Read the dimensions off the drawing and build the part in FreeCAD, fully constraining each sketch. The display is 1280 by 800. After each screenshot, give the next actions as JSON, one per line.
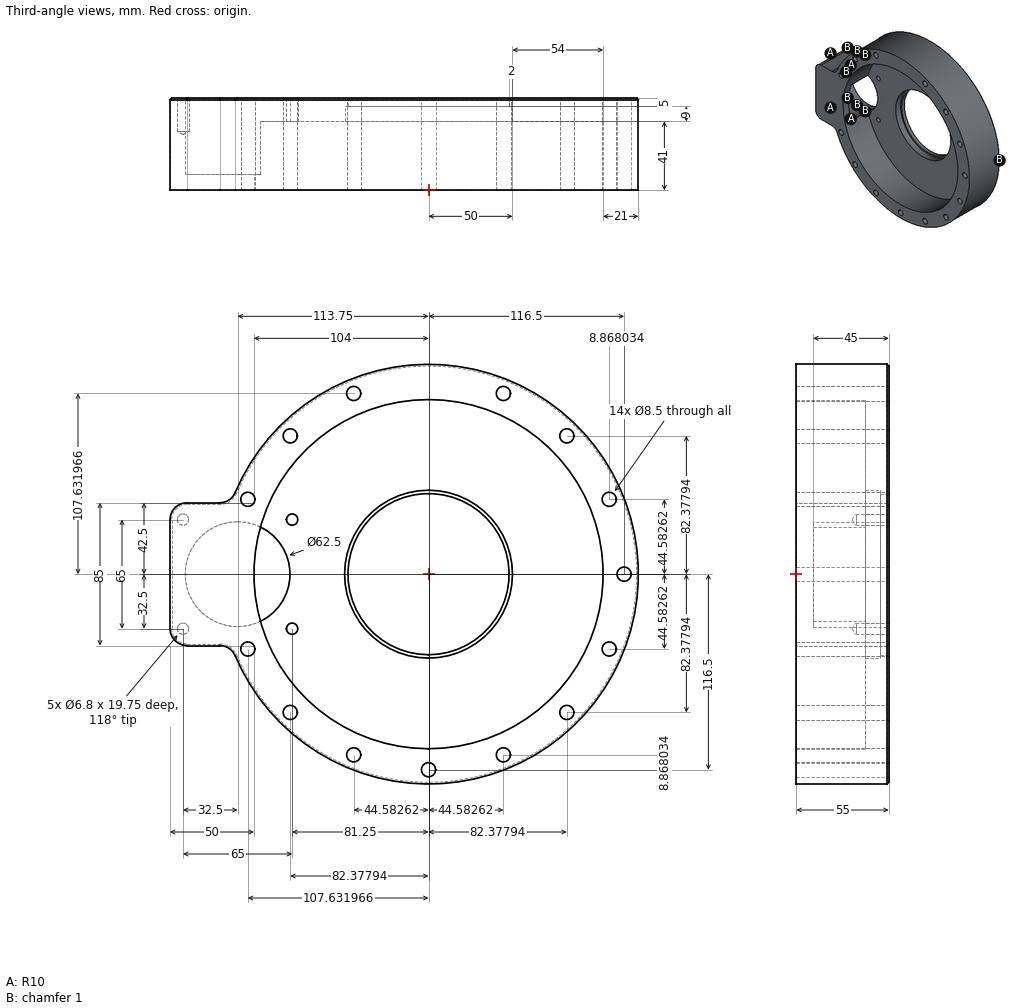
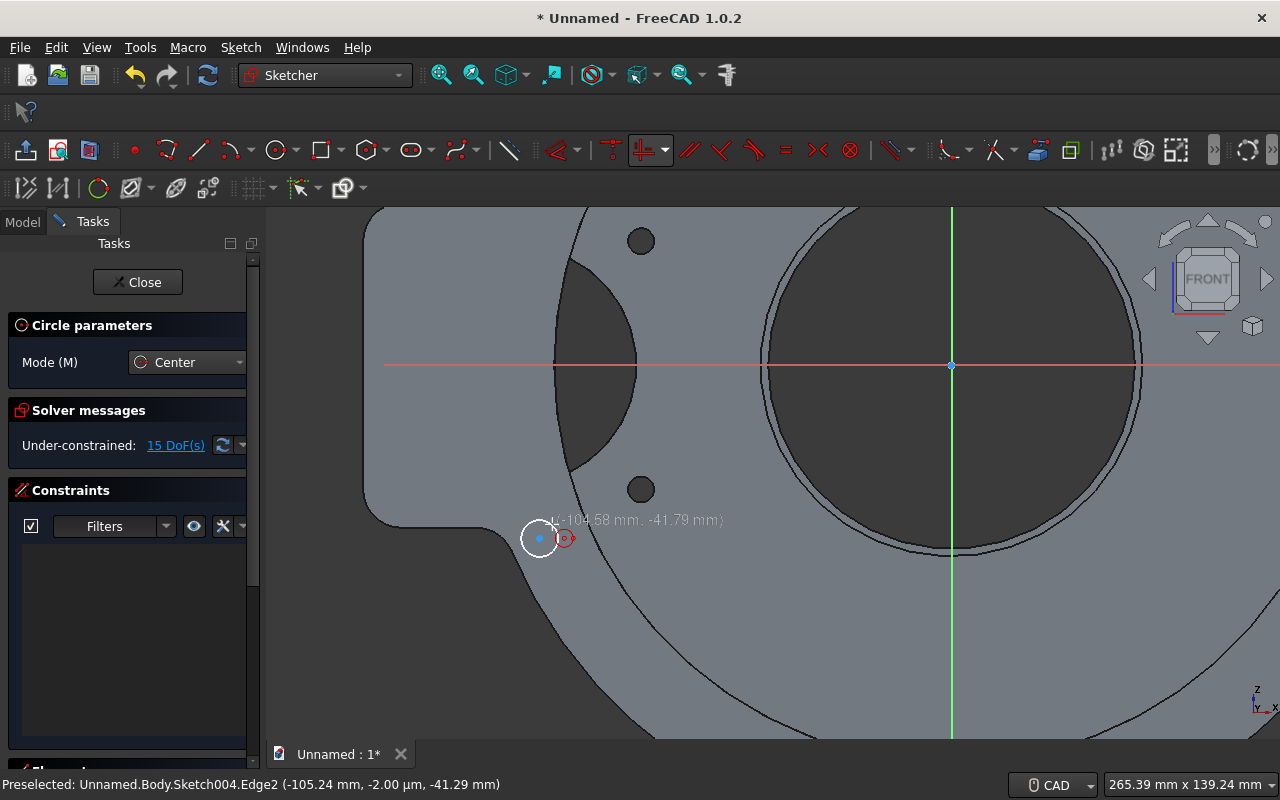
{"action": "scroll", "coordinate": [551, 526], "scroll_direction": "down", "scroll_amount": 5}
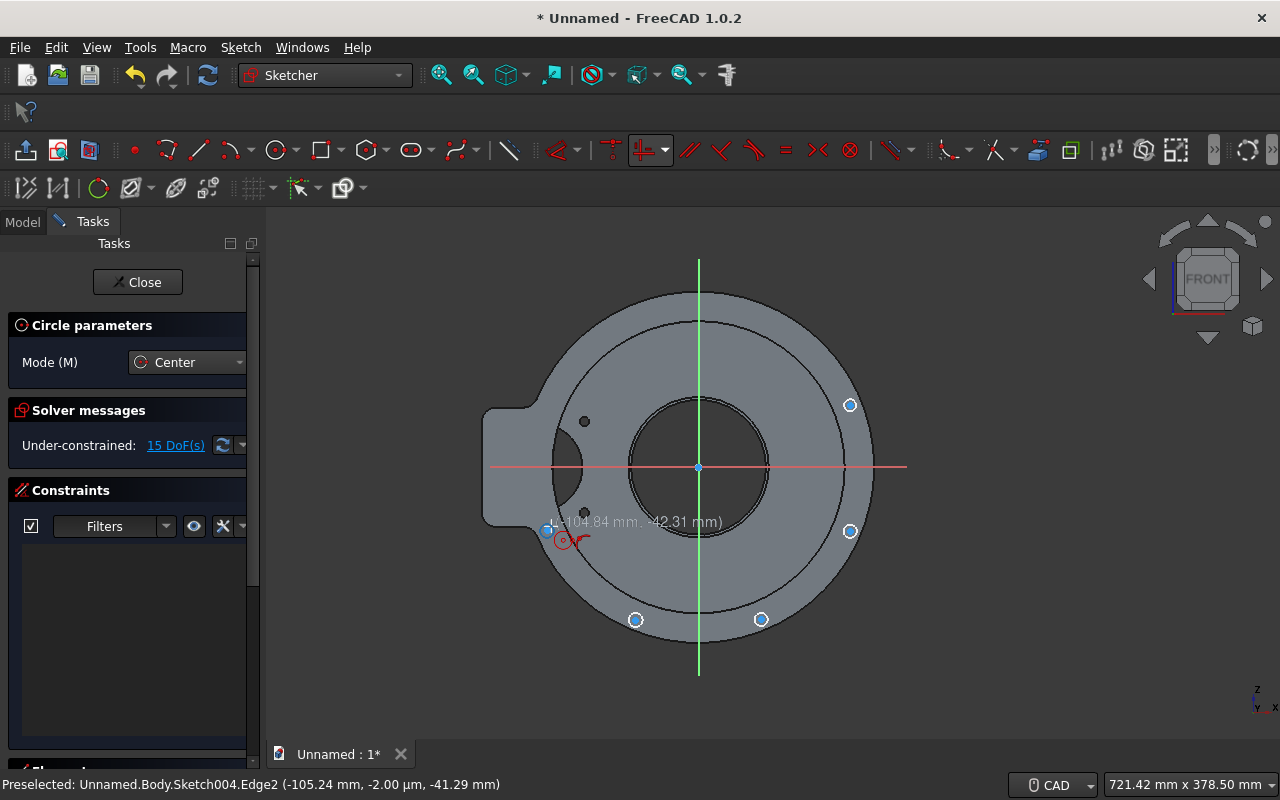
{"action": "scroll", "coordinate": [547, 405], "scroll_direction": "up", "scroll_amount": 7}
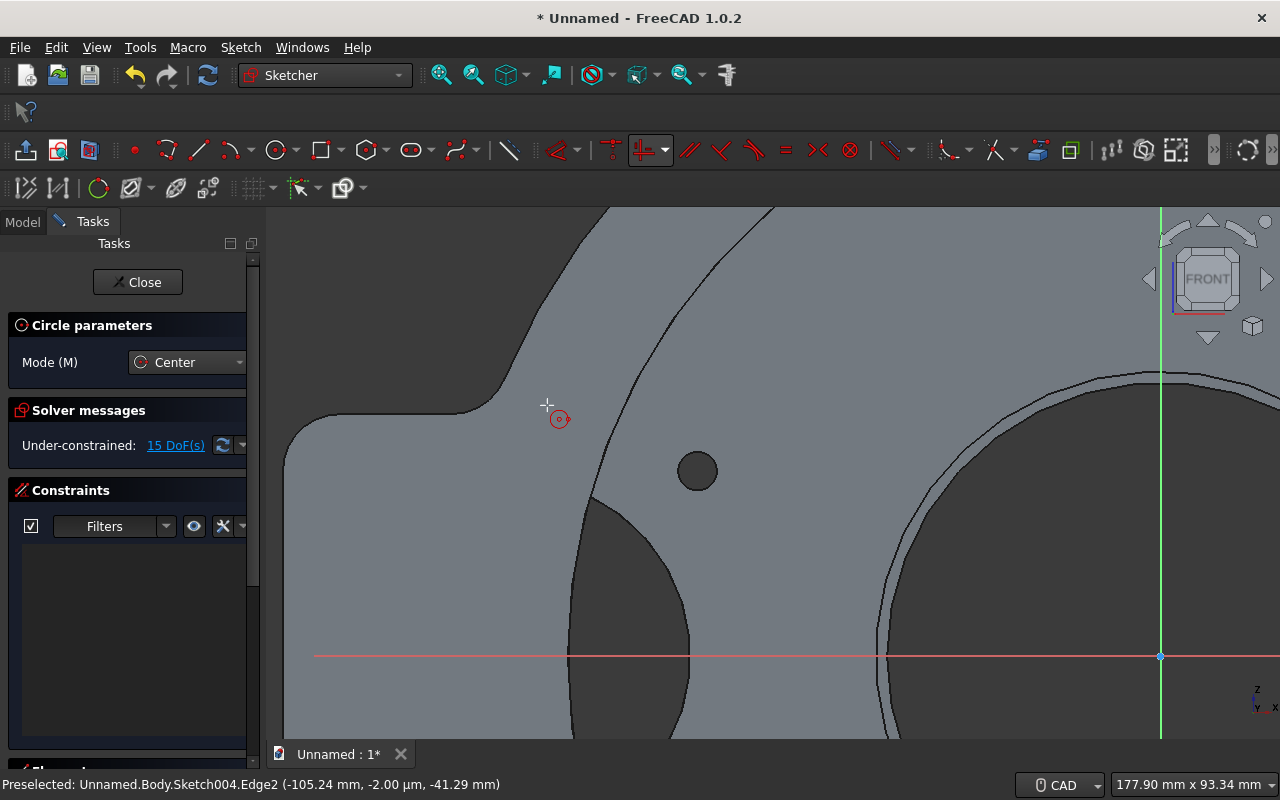
{"action": "scroll", "coordinate": [547, 405], "scroll_direction": "down", "scroll_amount": 7}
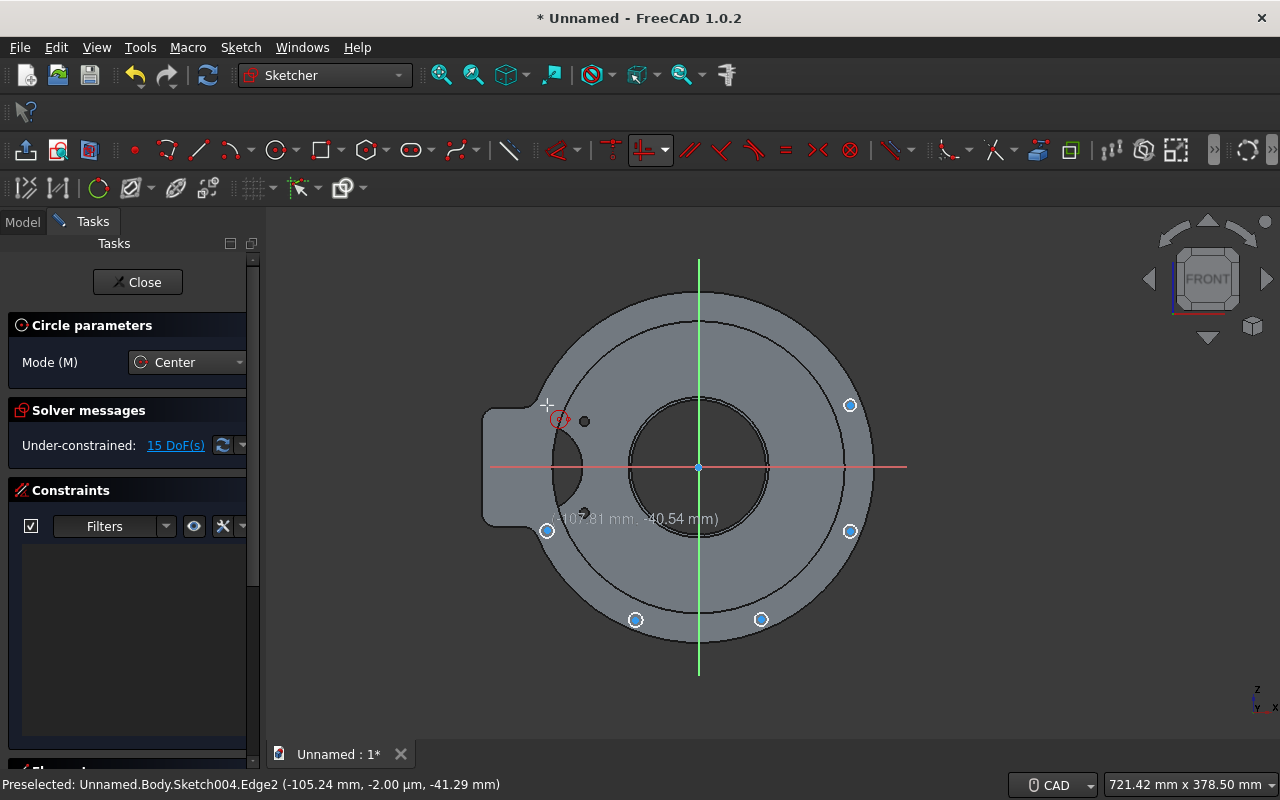
{"action": "left_click", "coordinate": [547, 405]}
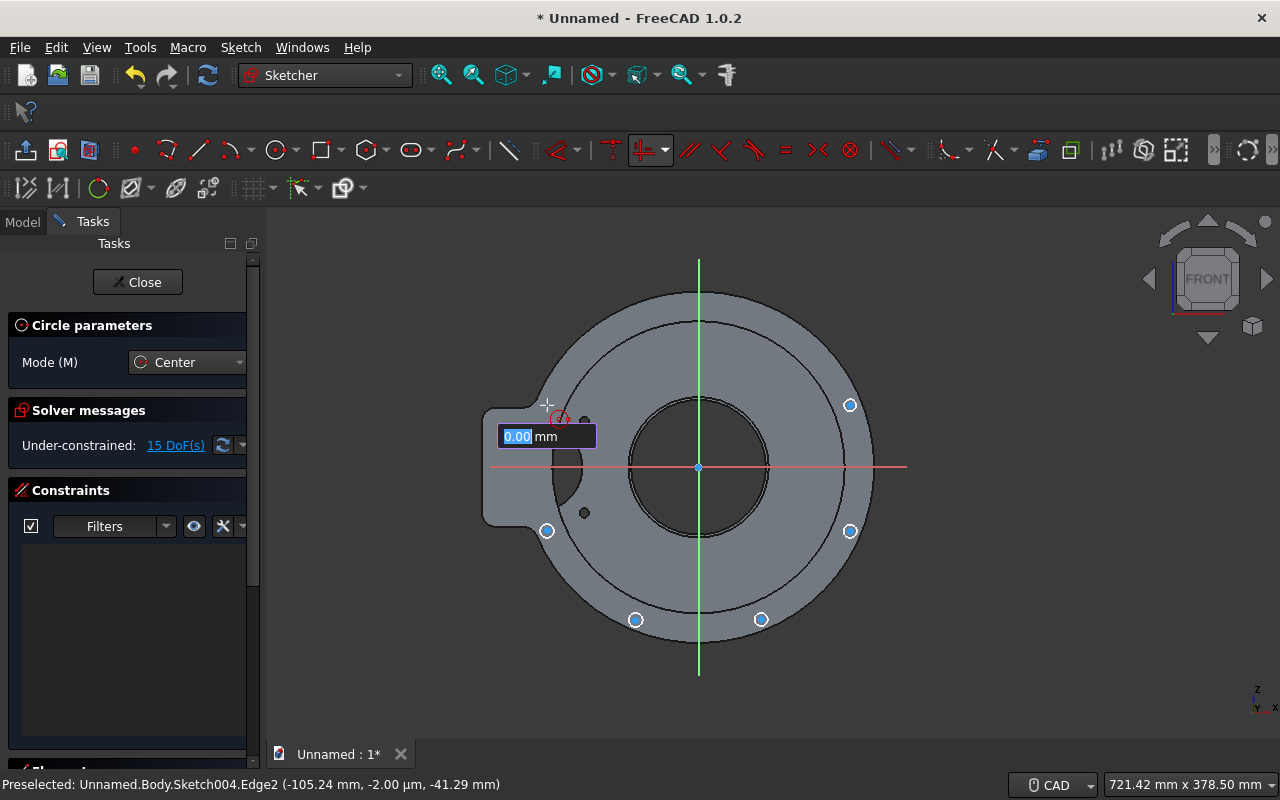
{"action": "scroll", "coordinate": [551, 400], "scroll_direction": "up", "scroll_amount": 5}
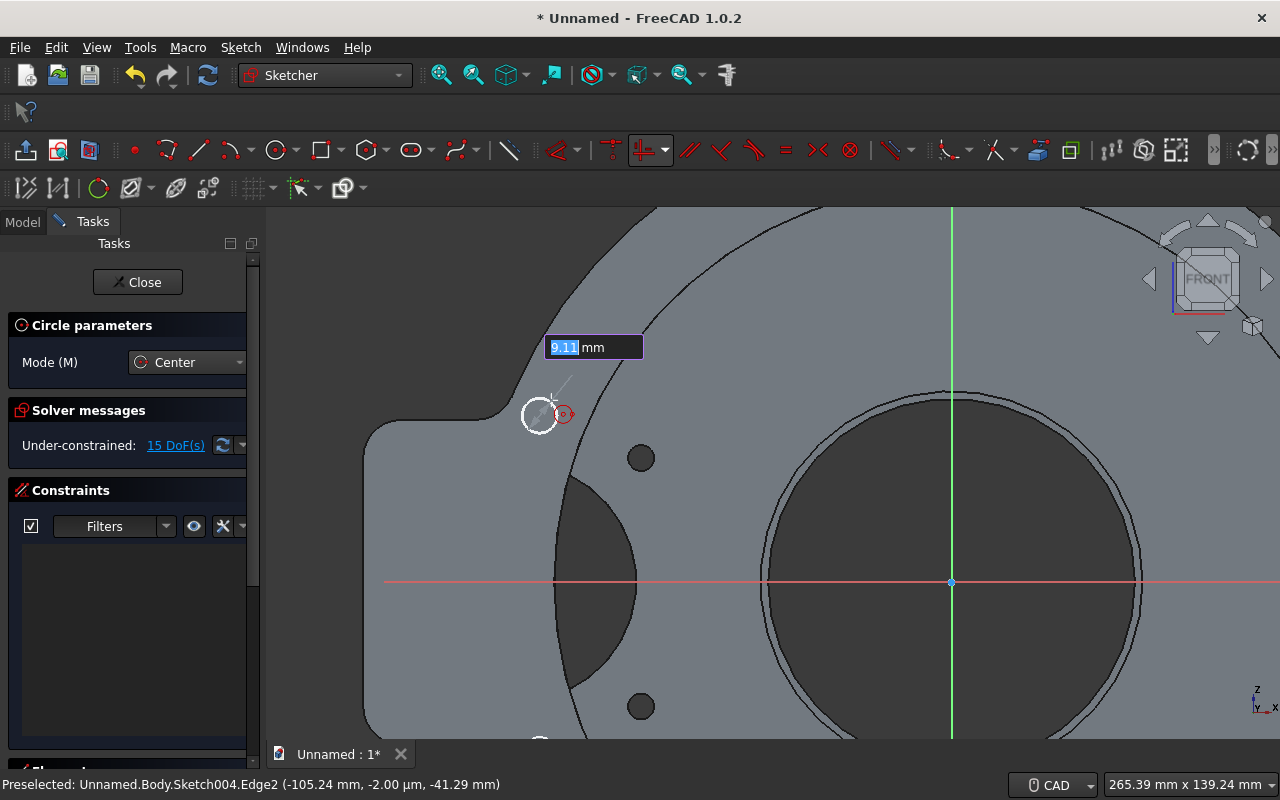
{"action": "left_click", "coordinate": [552, 400]}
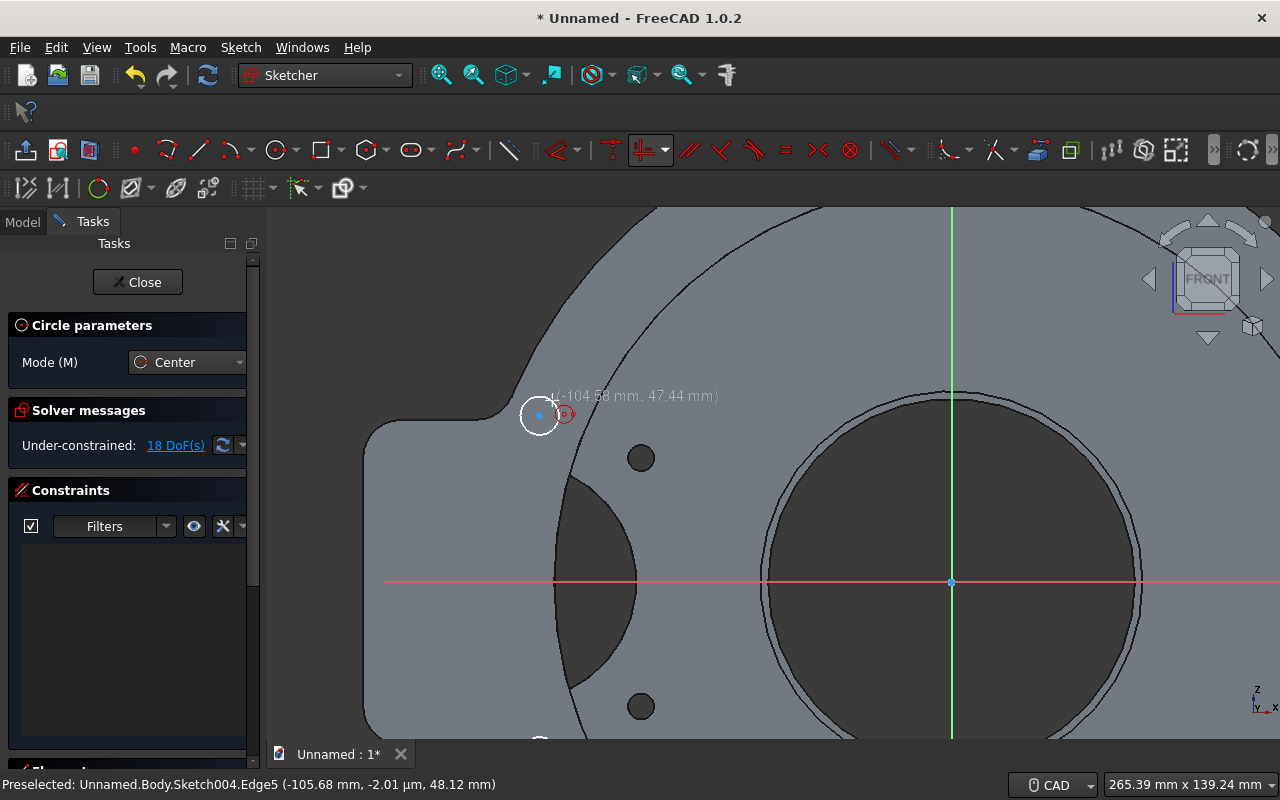
{"action": "scroll", "coordinate": [551, 400], "scroll_direction": "down", "scroll_amount": 5}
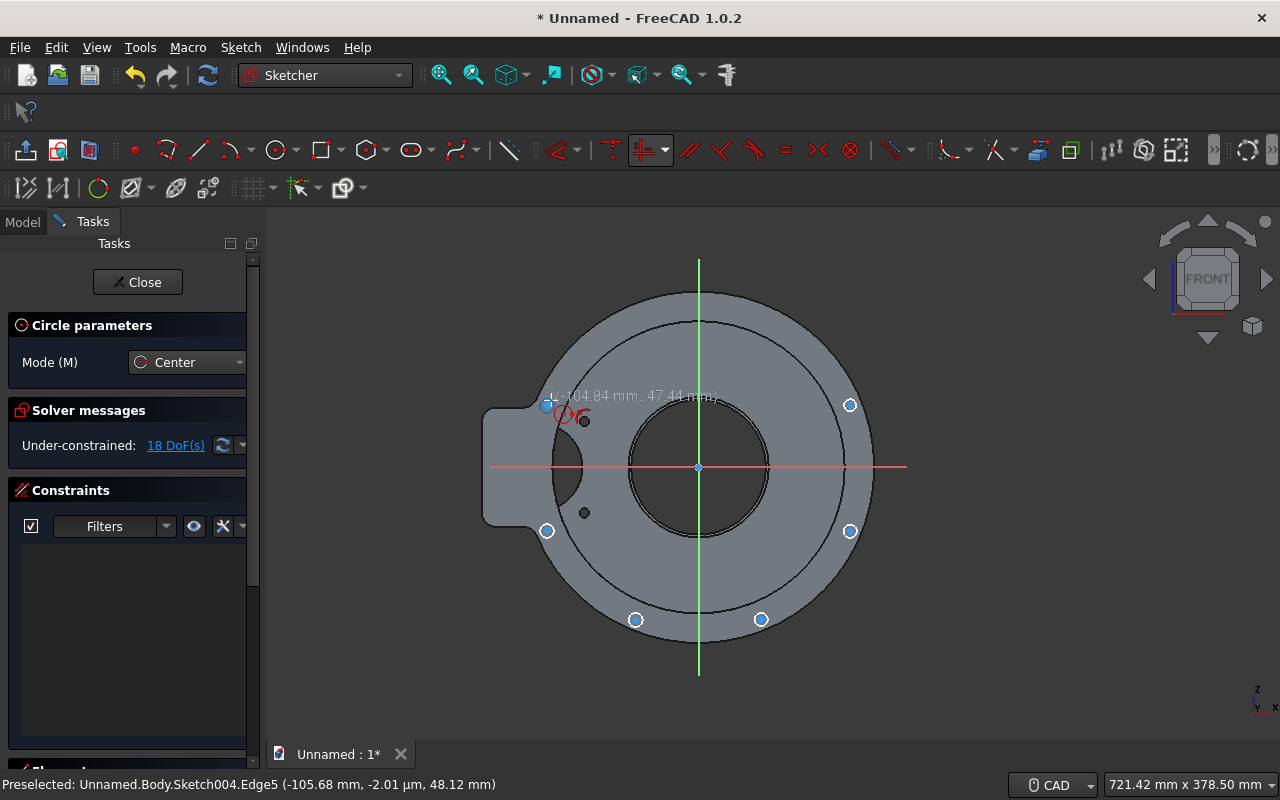
{"action": "scroll", "coordinate": [636, 316], "scroll_direction": "up", "scroll_amount": 7}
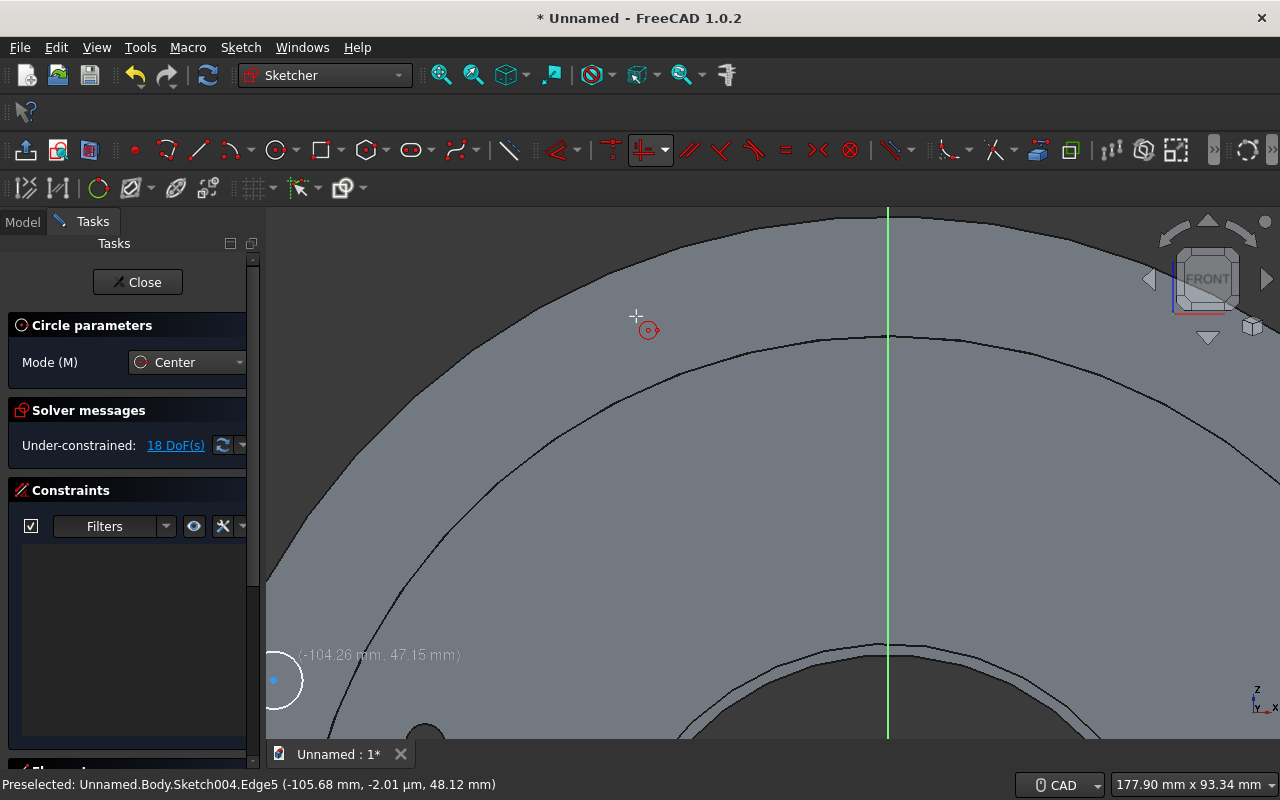
{"action": "scroll", "coordinate": [636, 316], "scroll_direction": "down", "scroll_amount": 7}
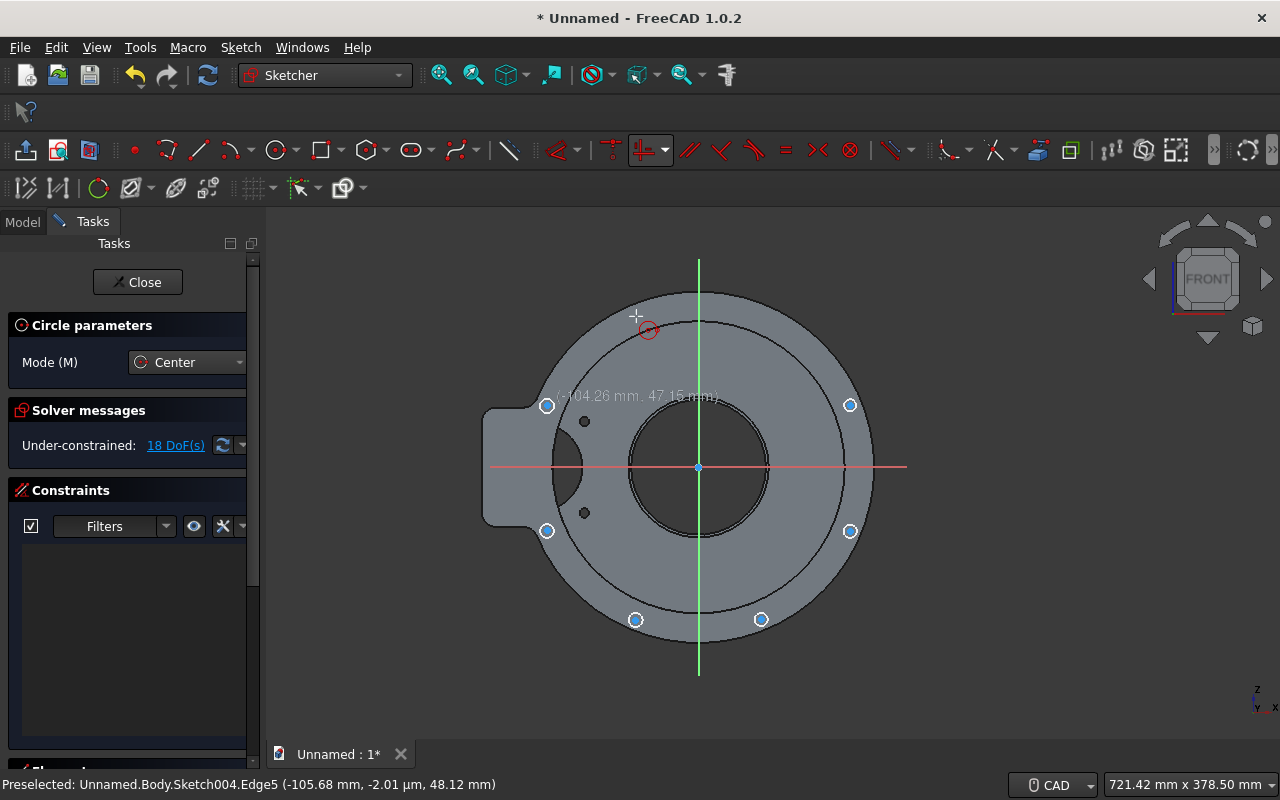
{"action": "left_click", "coordinate": [636, 316]}